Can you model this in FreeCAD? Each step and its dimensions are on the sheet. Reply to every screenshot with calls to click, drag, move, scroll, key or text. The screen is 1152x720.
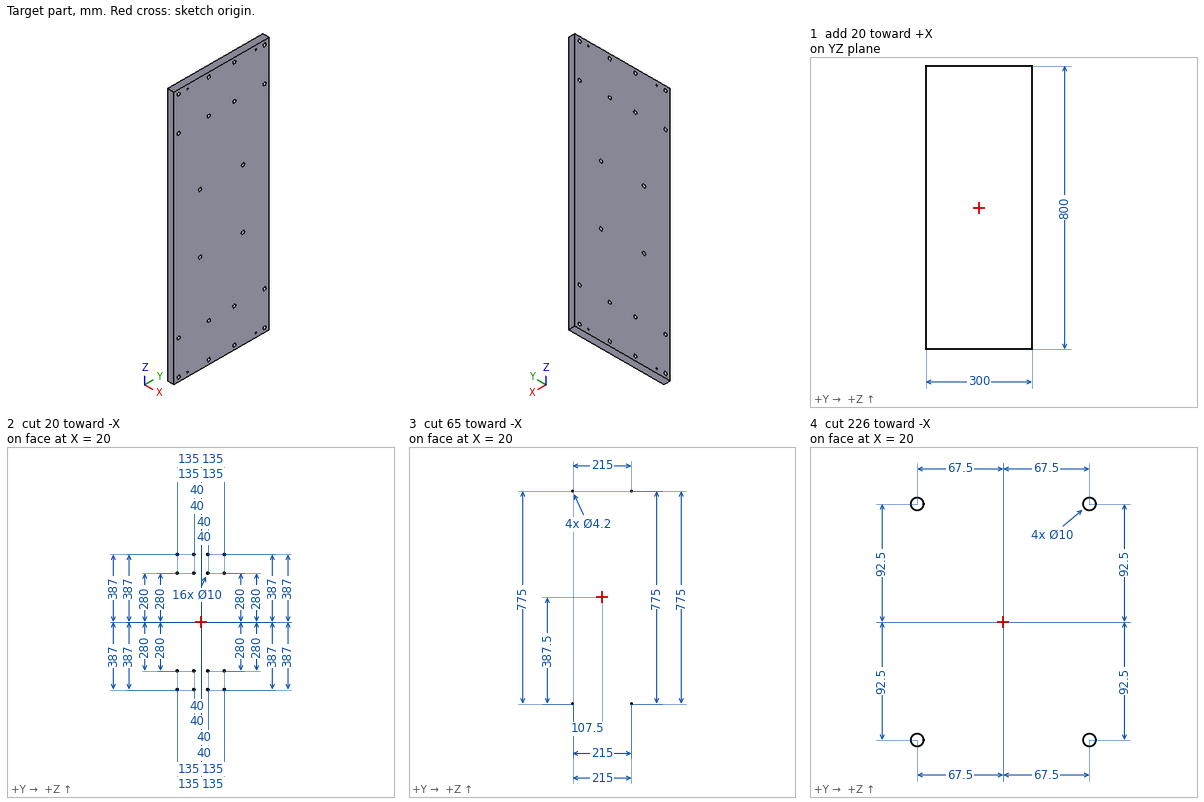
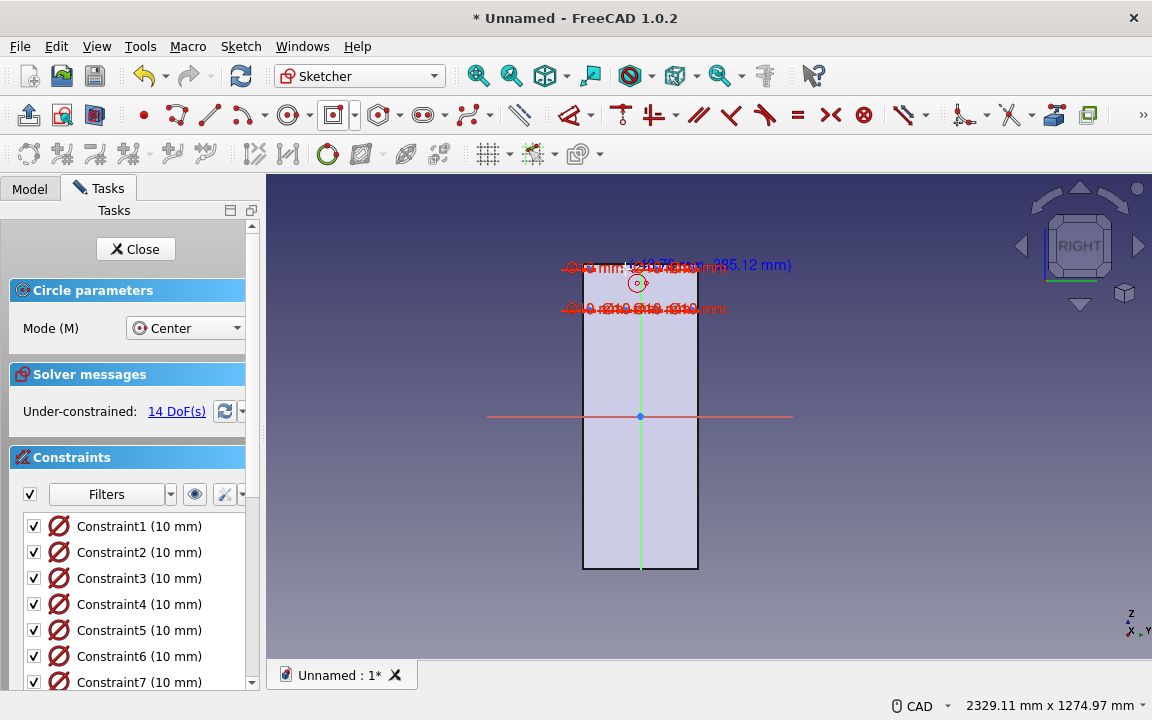
click(625, 269)
move(624, 268)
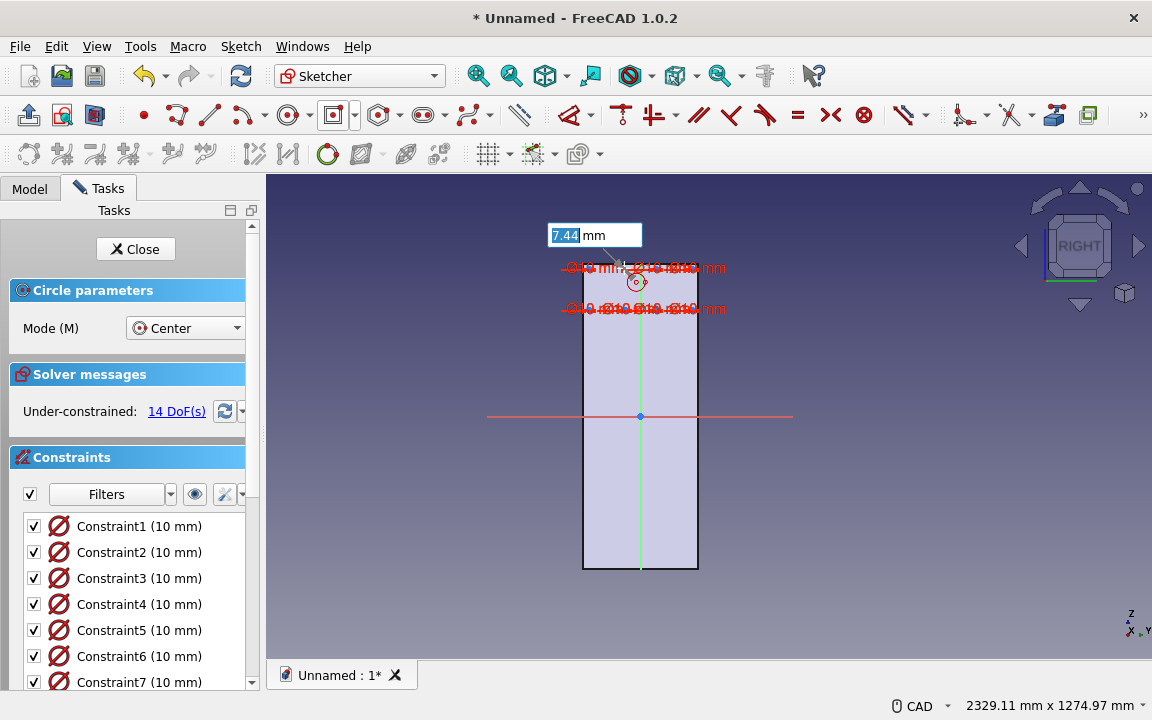
text(10)
key(Return)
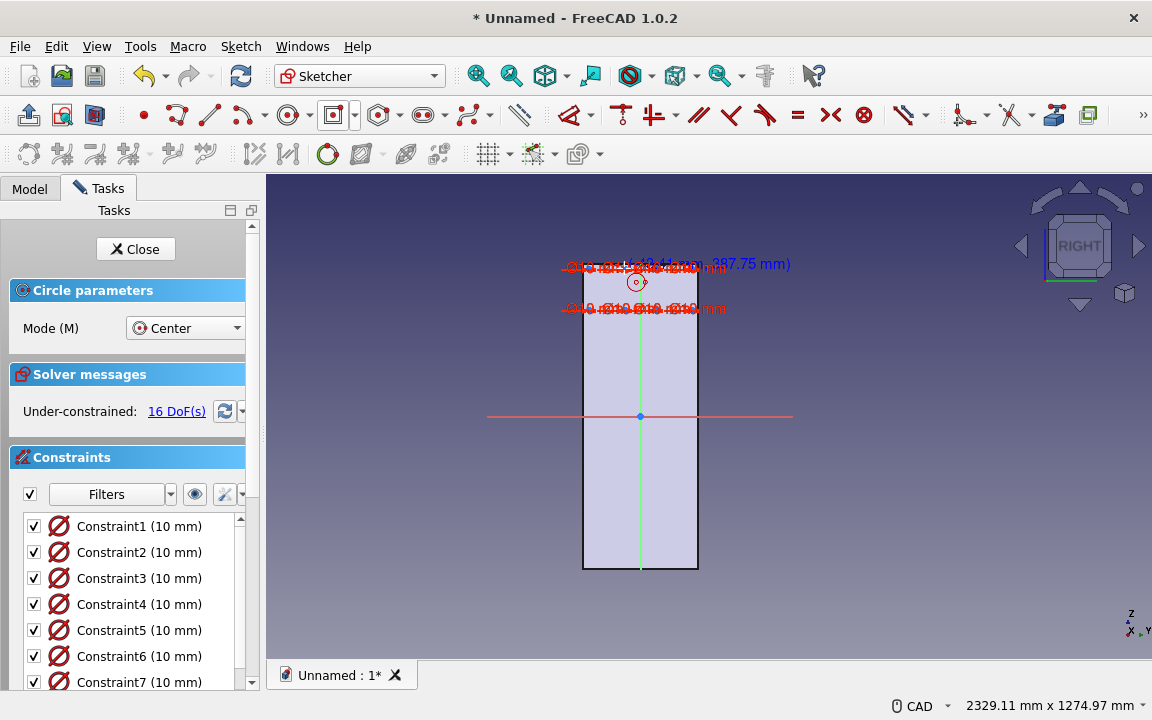
scroll(625, 523, up, 13)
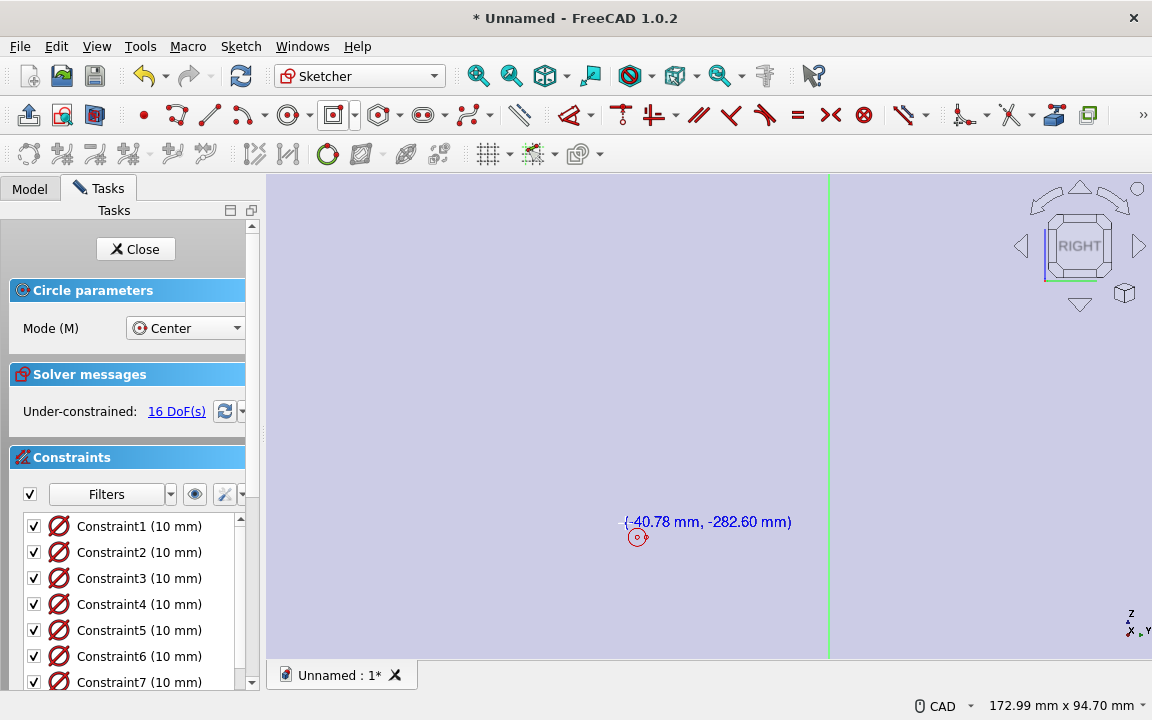
scroll(625, 524, down, 13)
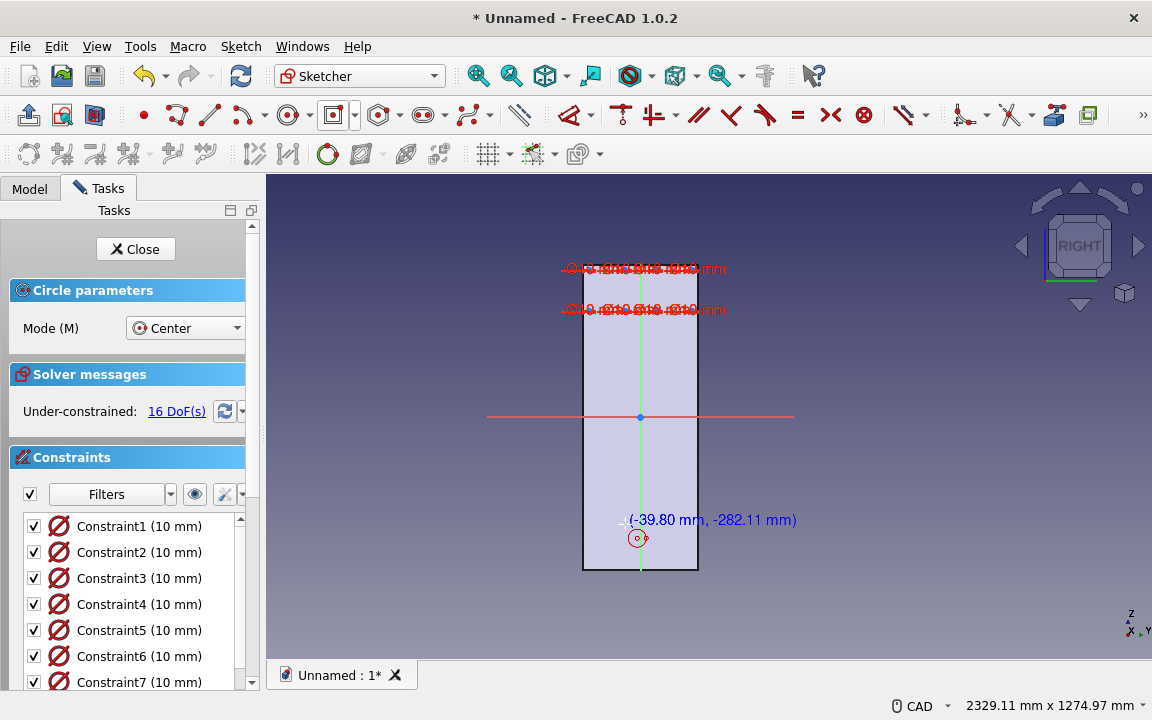
click(625, 524)
move(624, 523)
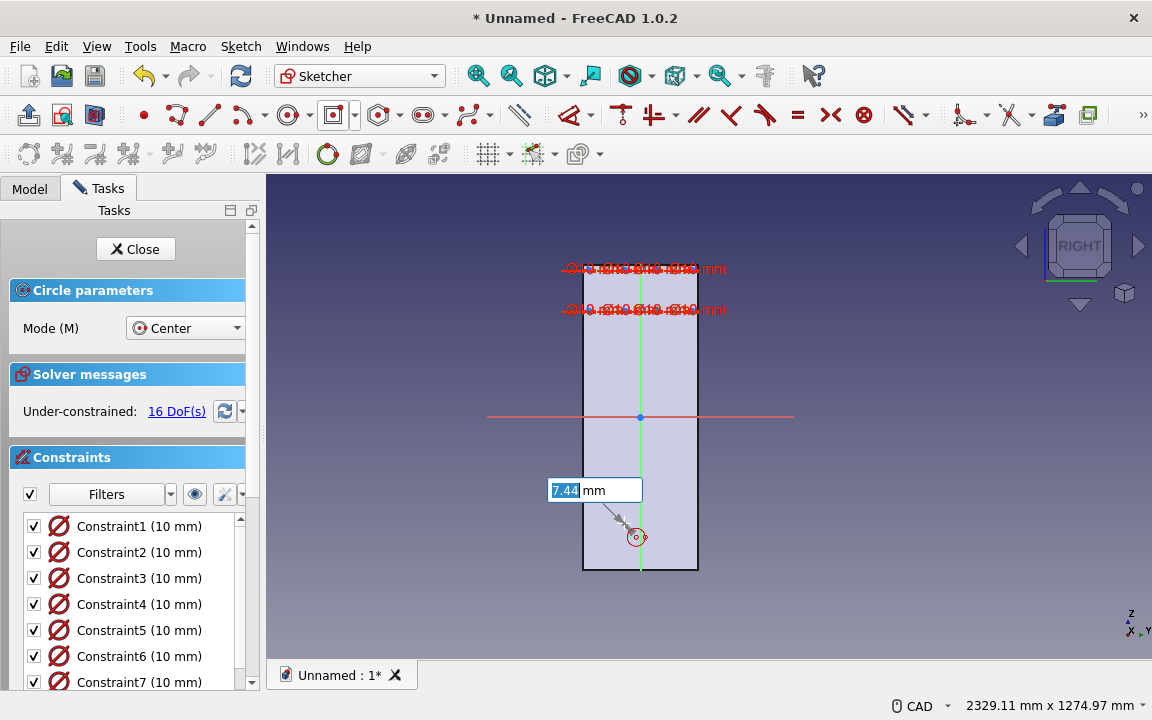
text(10)
key(Return)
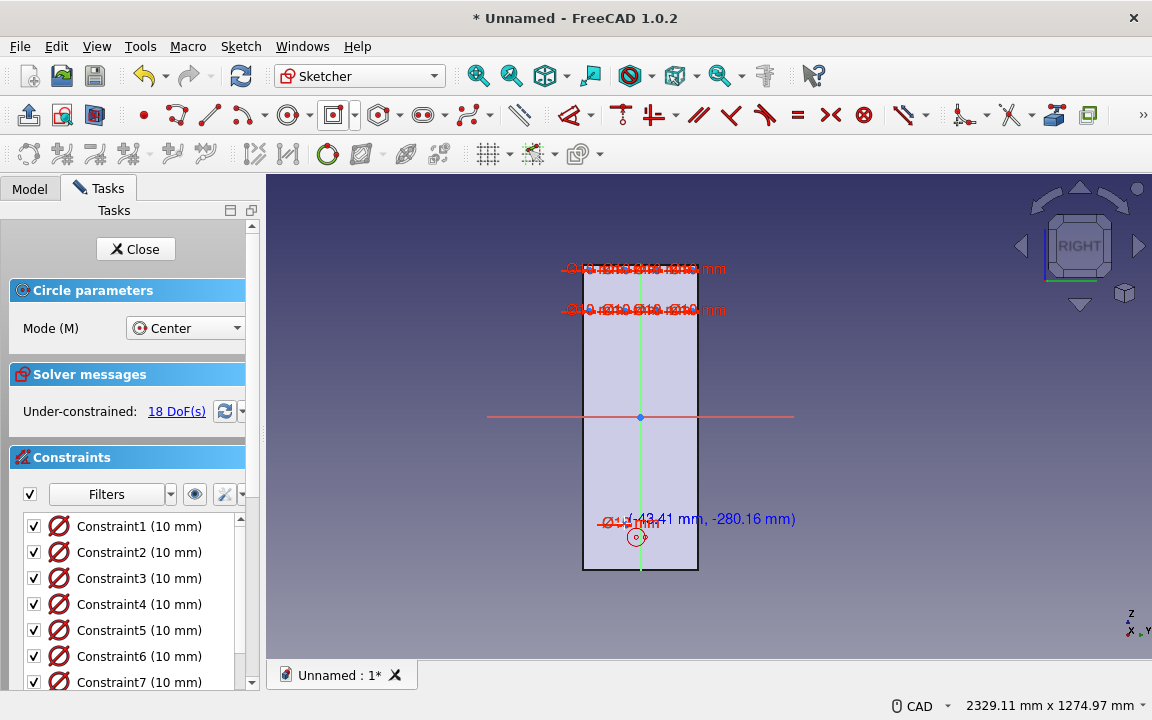
scroll(589, 524, up, 13)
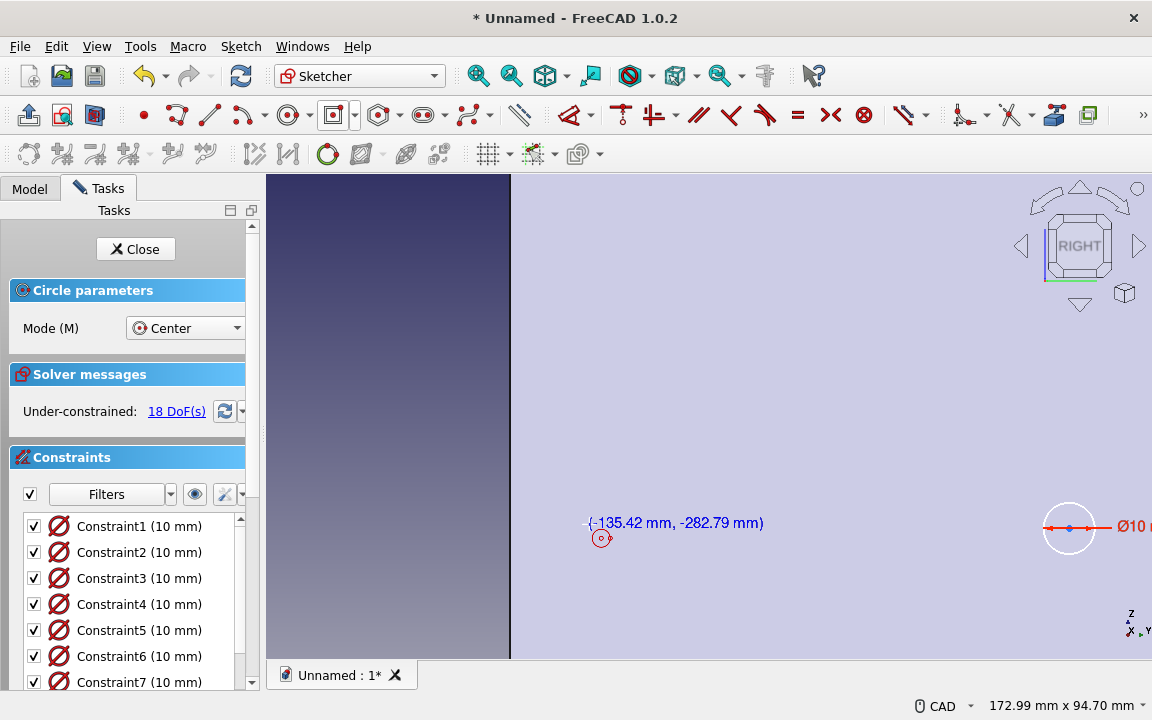
scroll(589, 524, down, 13)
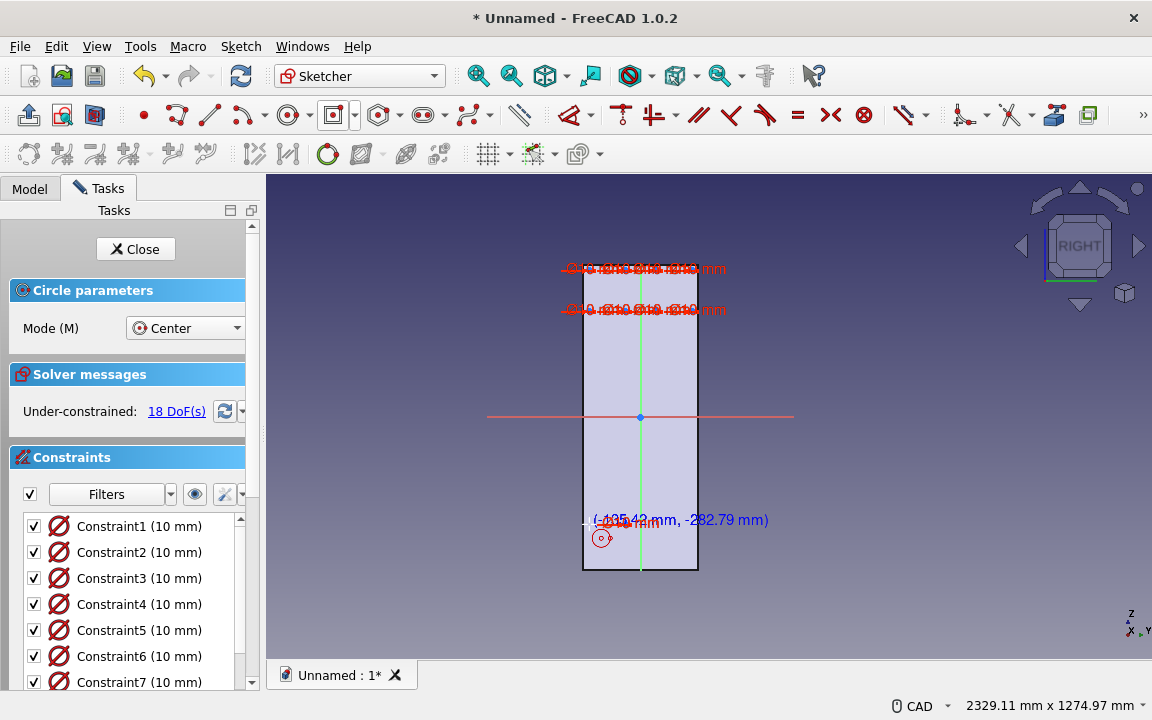
click(589, 524)
move(591, 523)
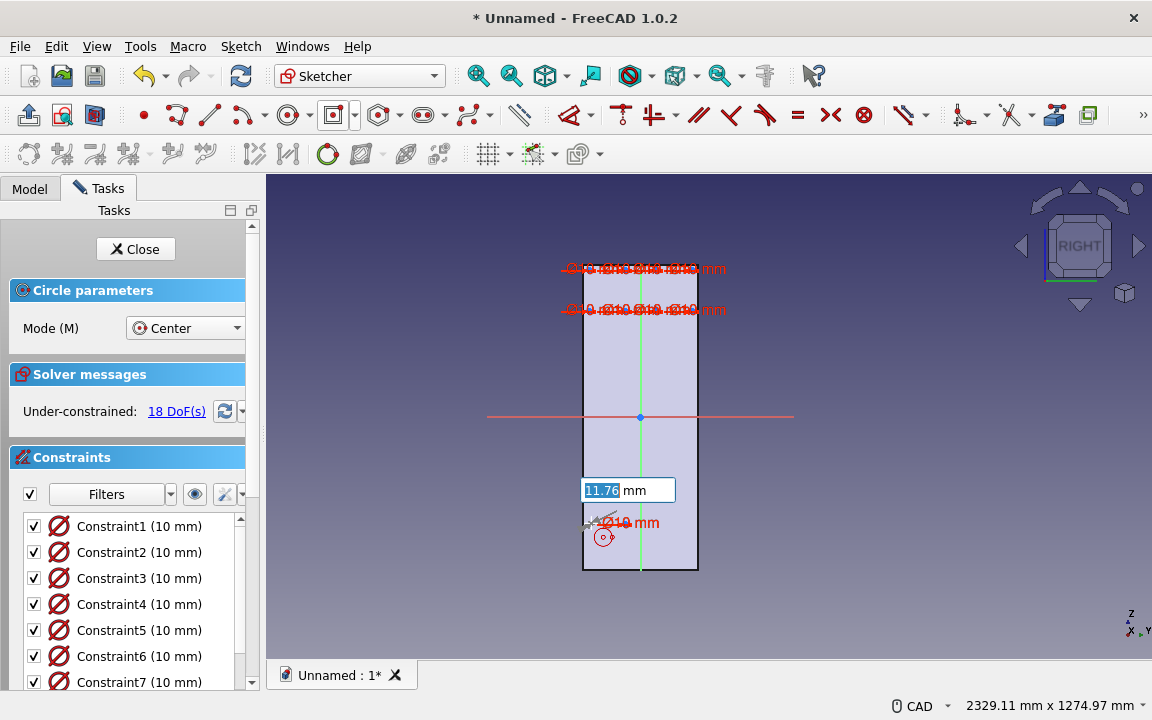
text(10)
key(Return)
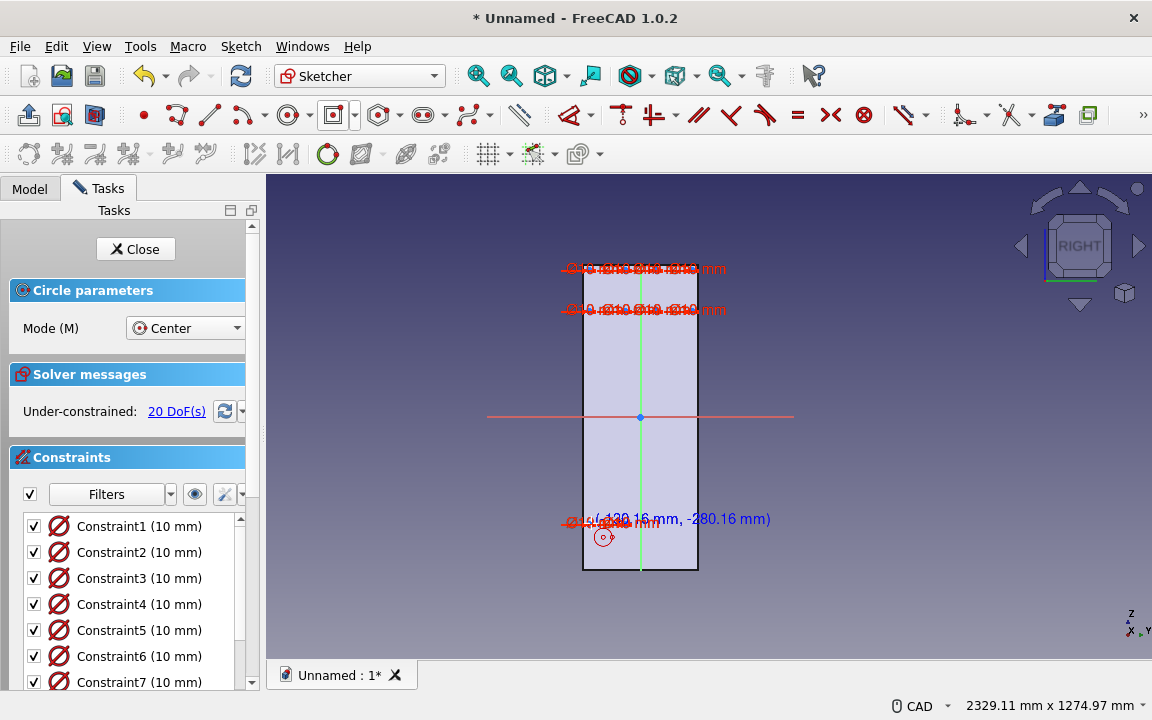
scroll(589, 565, up, 13)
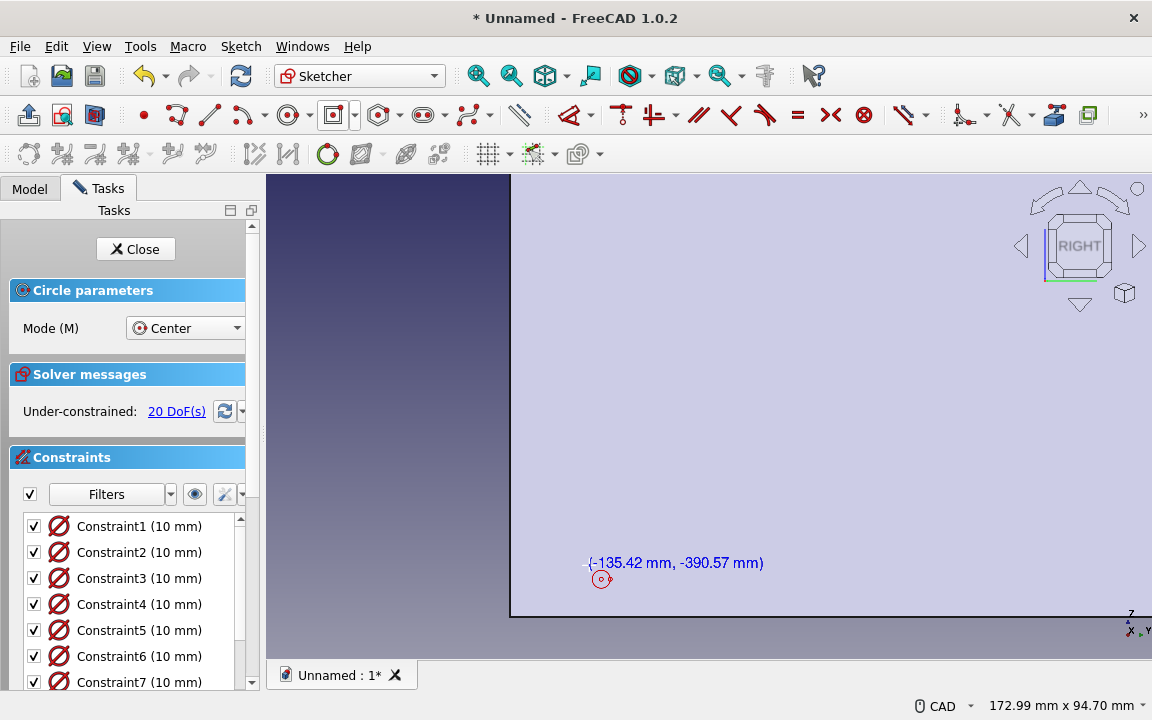
scroll(589, 565, down, 13)